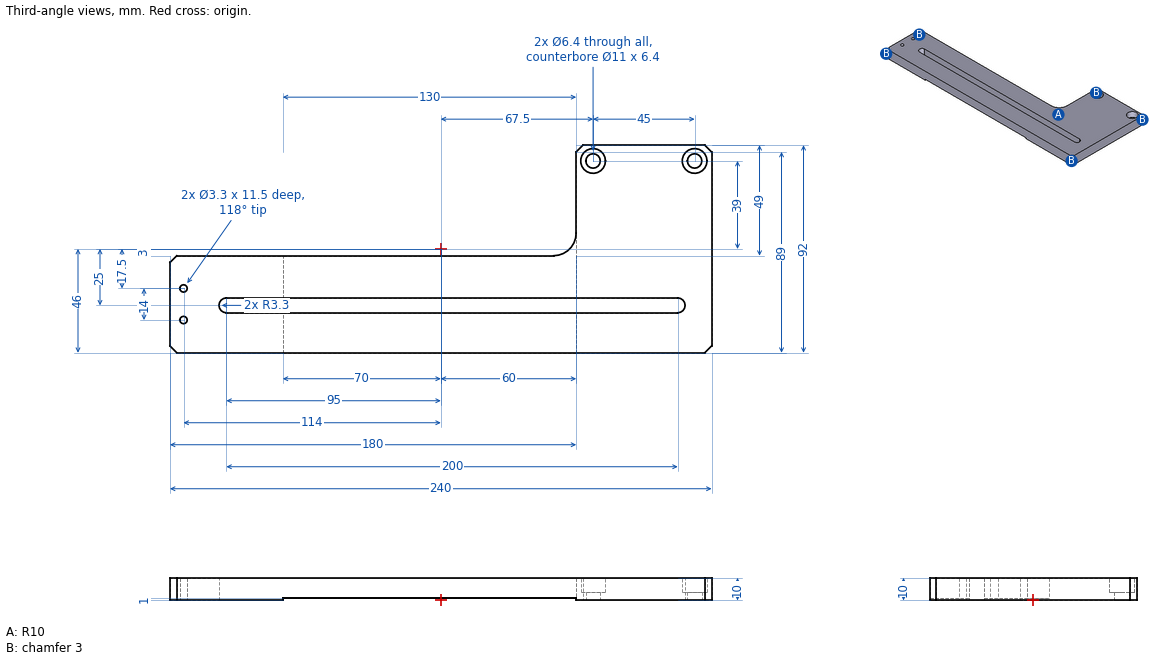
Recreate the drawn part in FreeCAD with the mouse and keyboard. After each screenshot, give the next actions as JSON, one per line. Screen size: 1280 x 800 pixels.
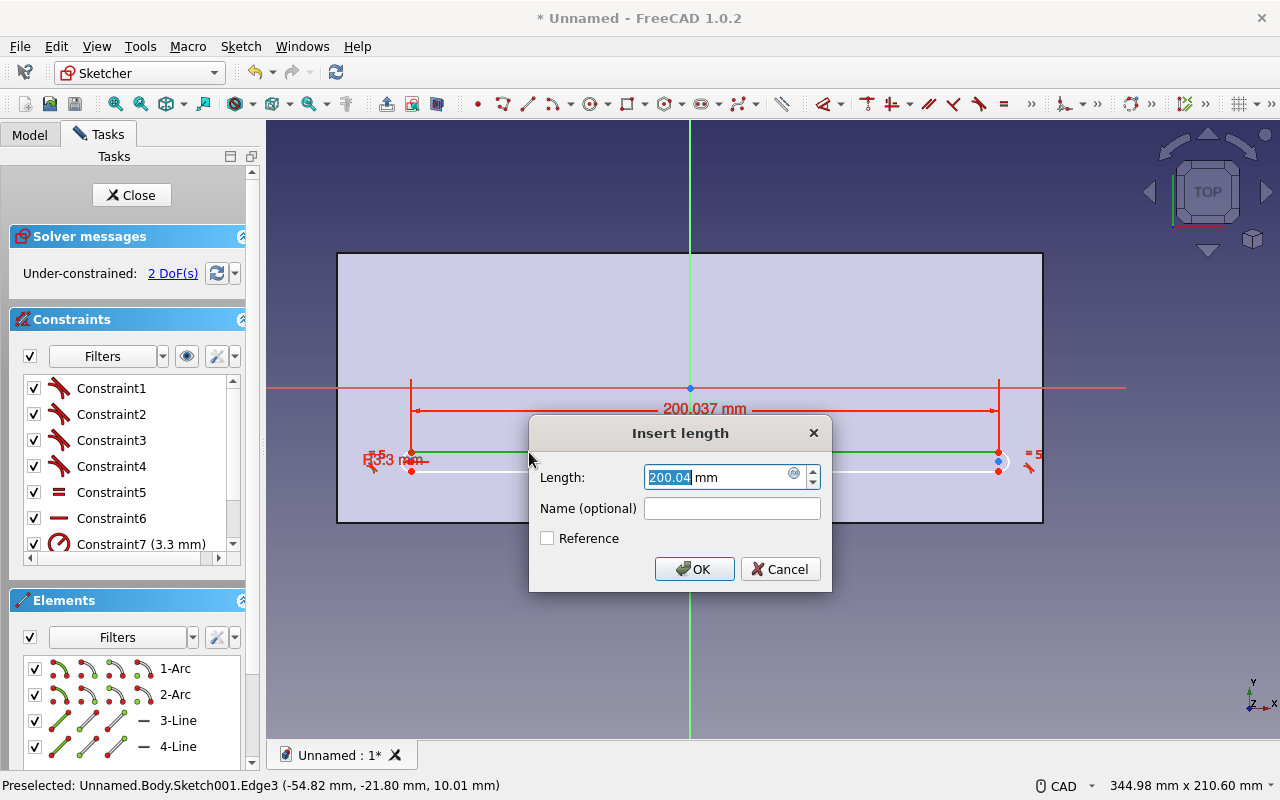
{"action": "type", "text": "200"}
{"action": "key", "text": "Return"}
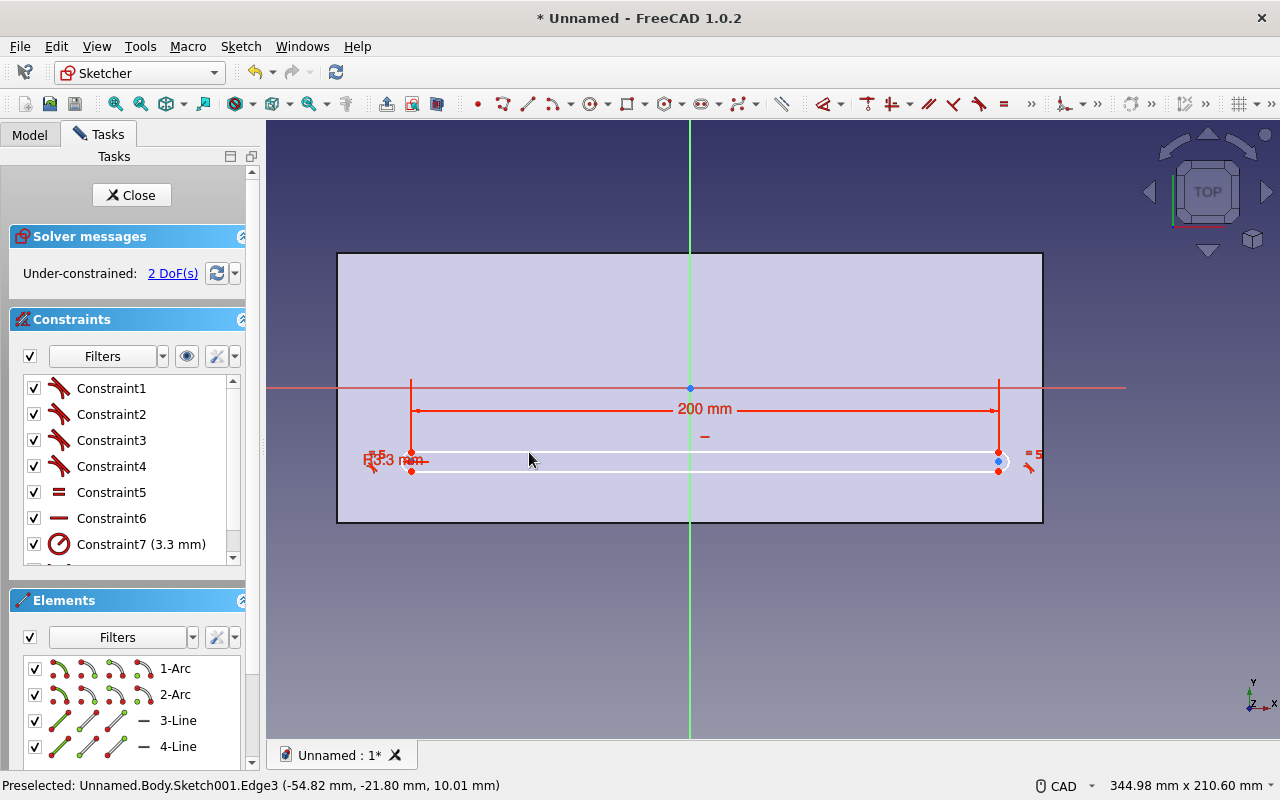
{"action": "scroll", "coordinate": [411, 452], "scroll_direction": "up", "scroll_amount": 2}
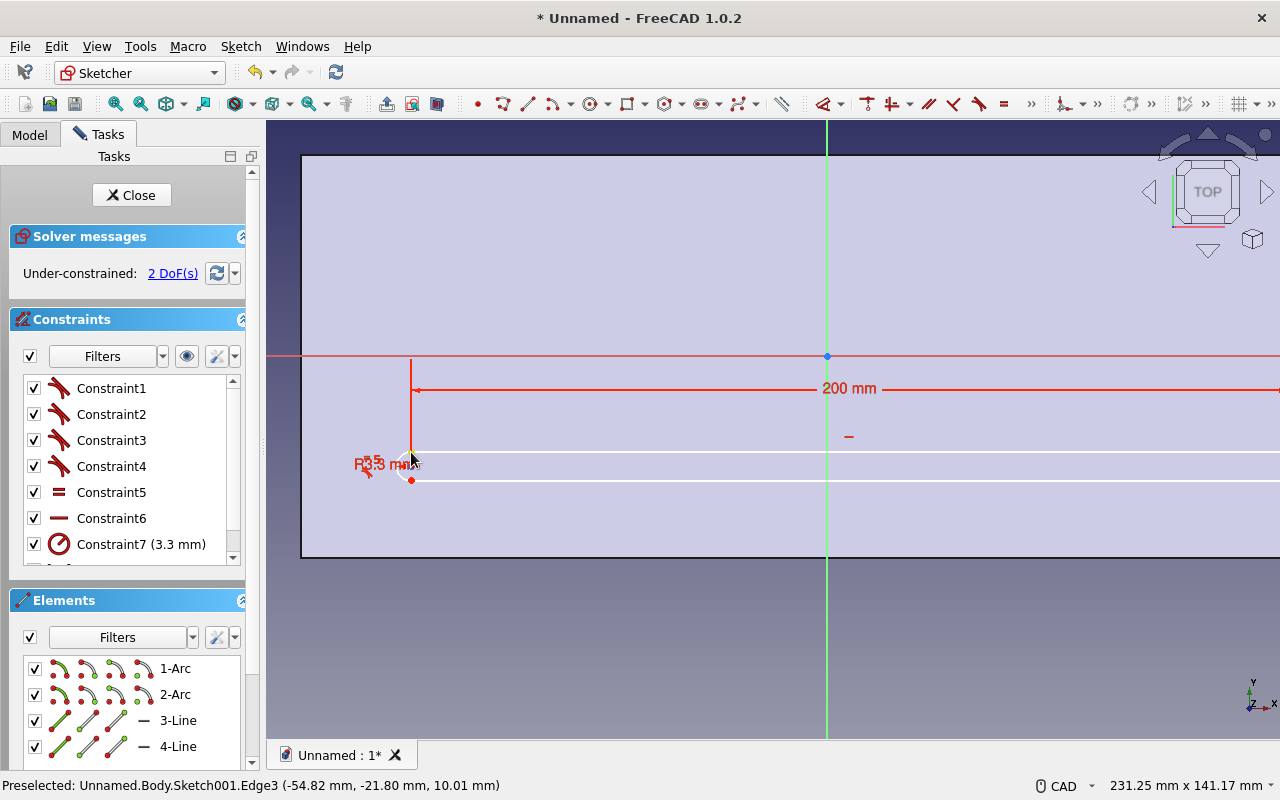
{"action": "left_click", "coordinate": [411, 452]}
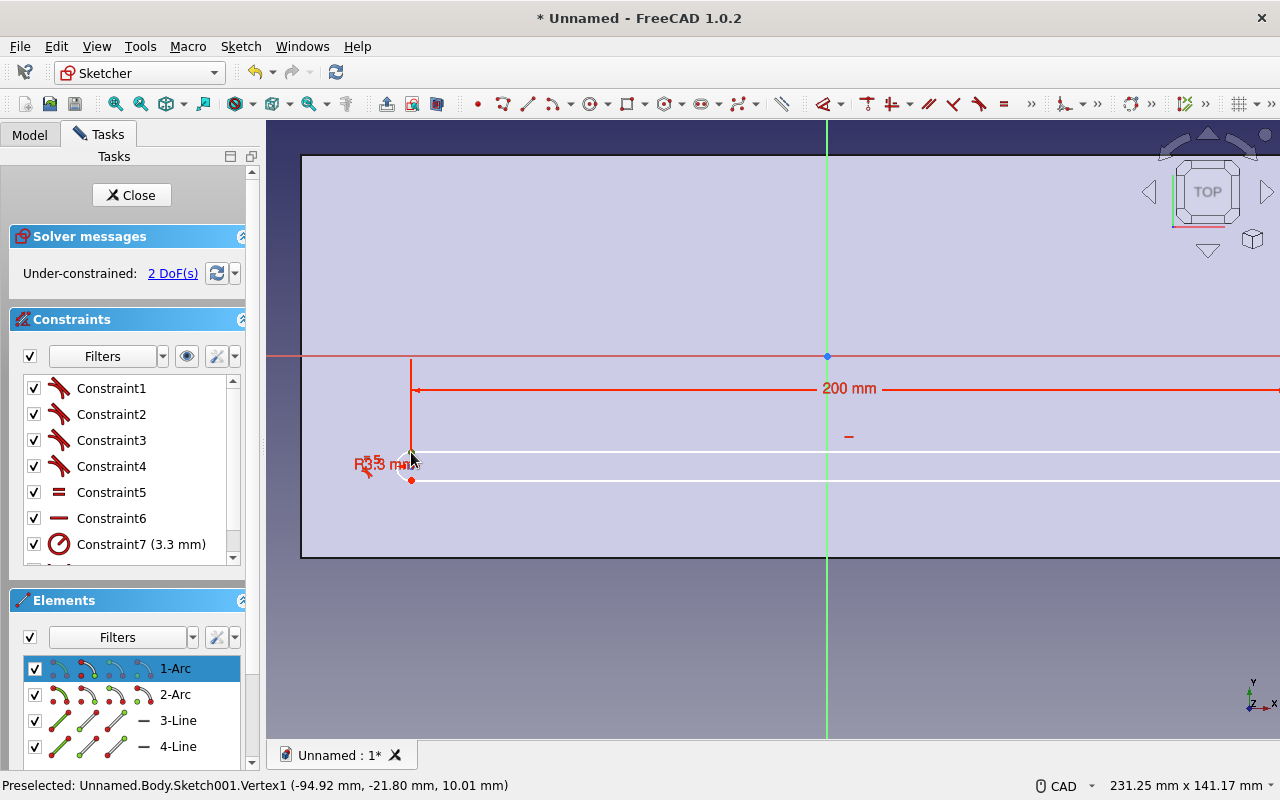
{"action": "key", "text": "l"}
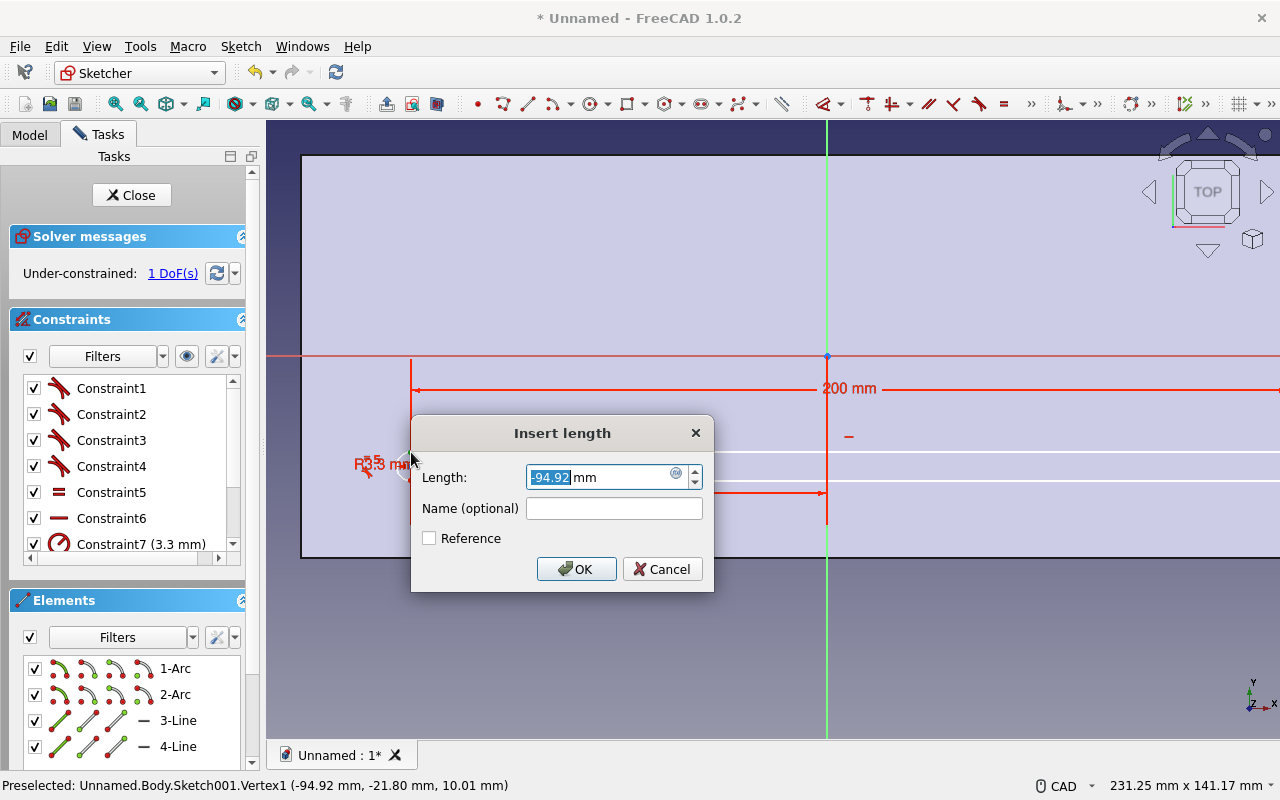
{"action": "type", "text": "-95"}
{"action": "key", "text": "Return"}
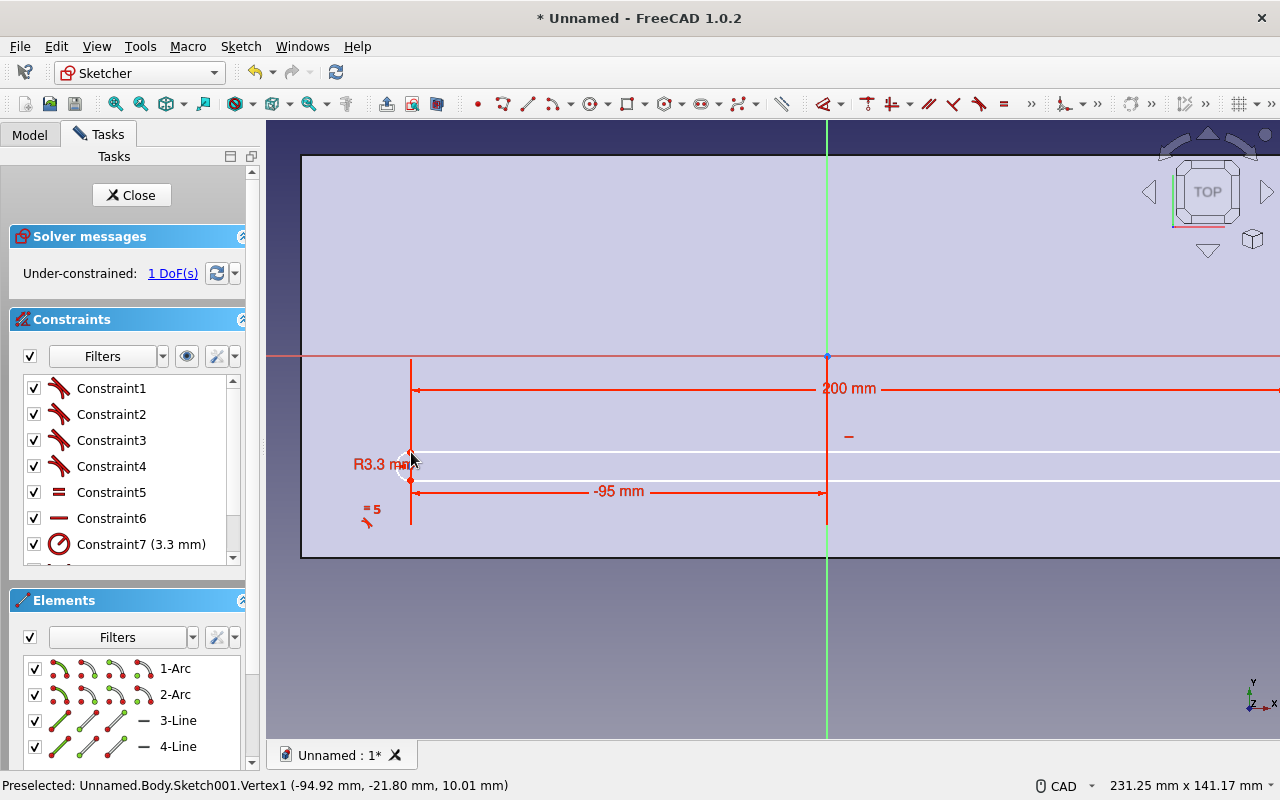
{"action": "left_click", "coordinate": [411, 466]}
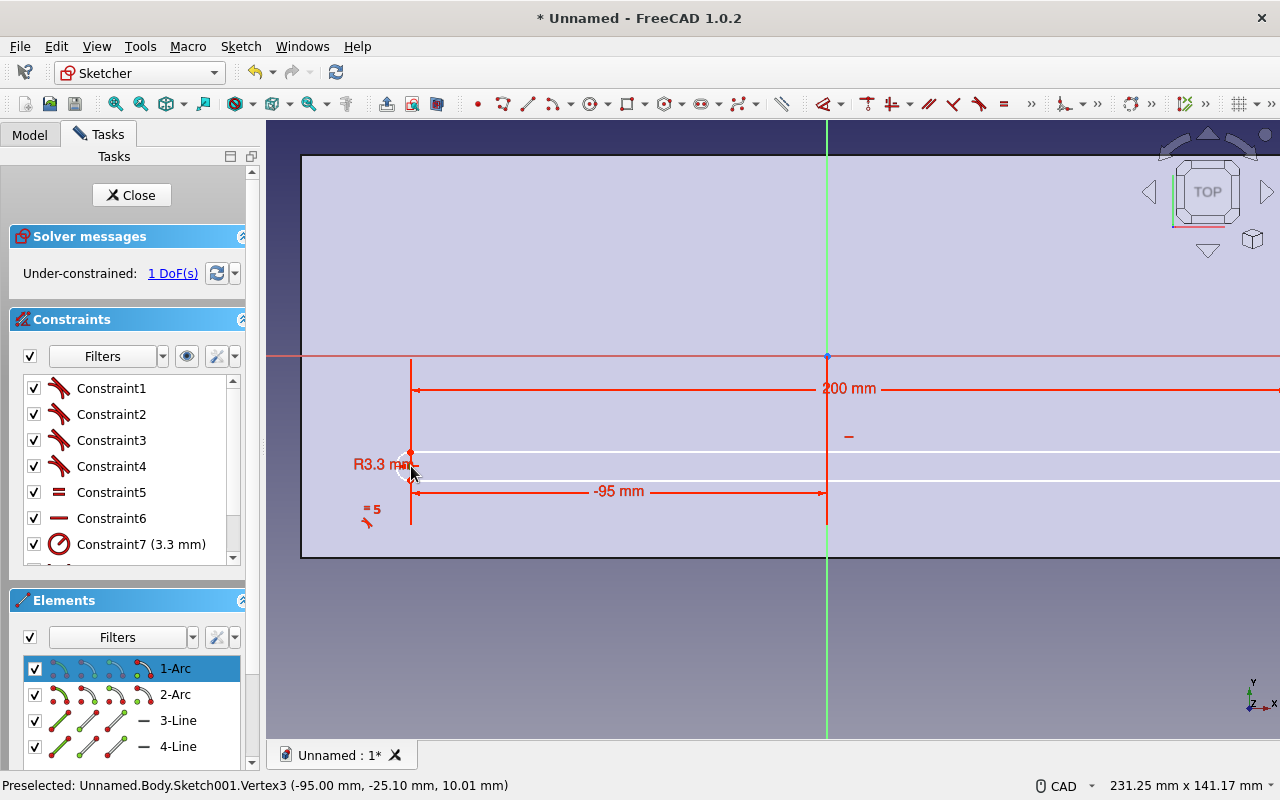
{"action": "key", "text": "i"}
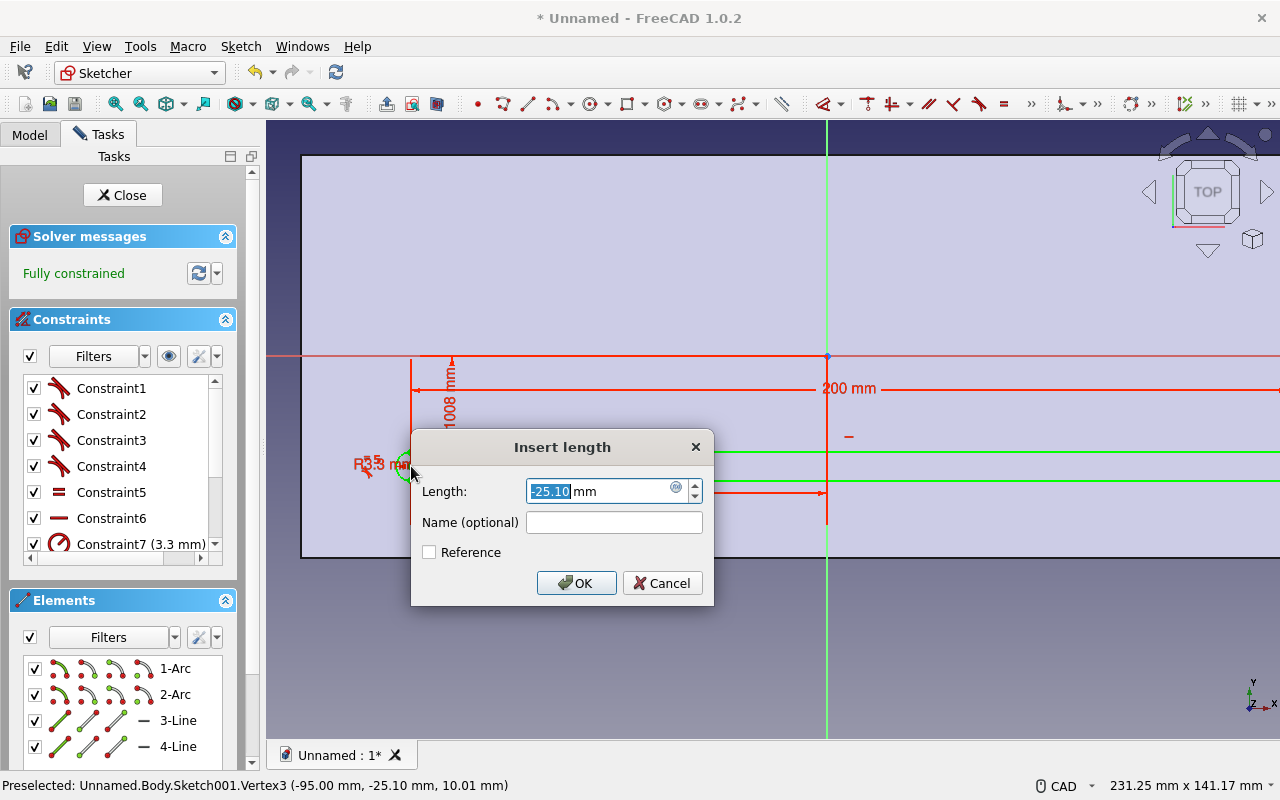
{"action": "type", "text": "-25"}
{"action": "key", "text": "Return"}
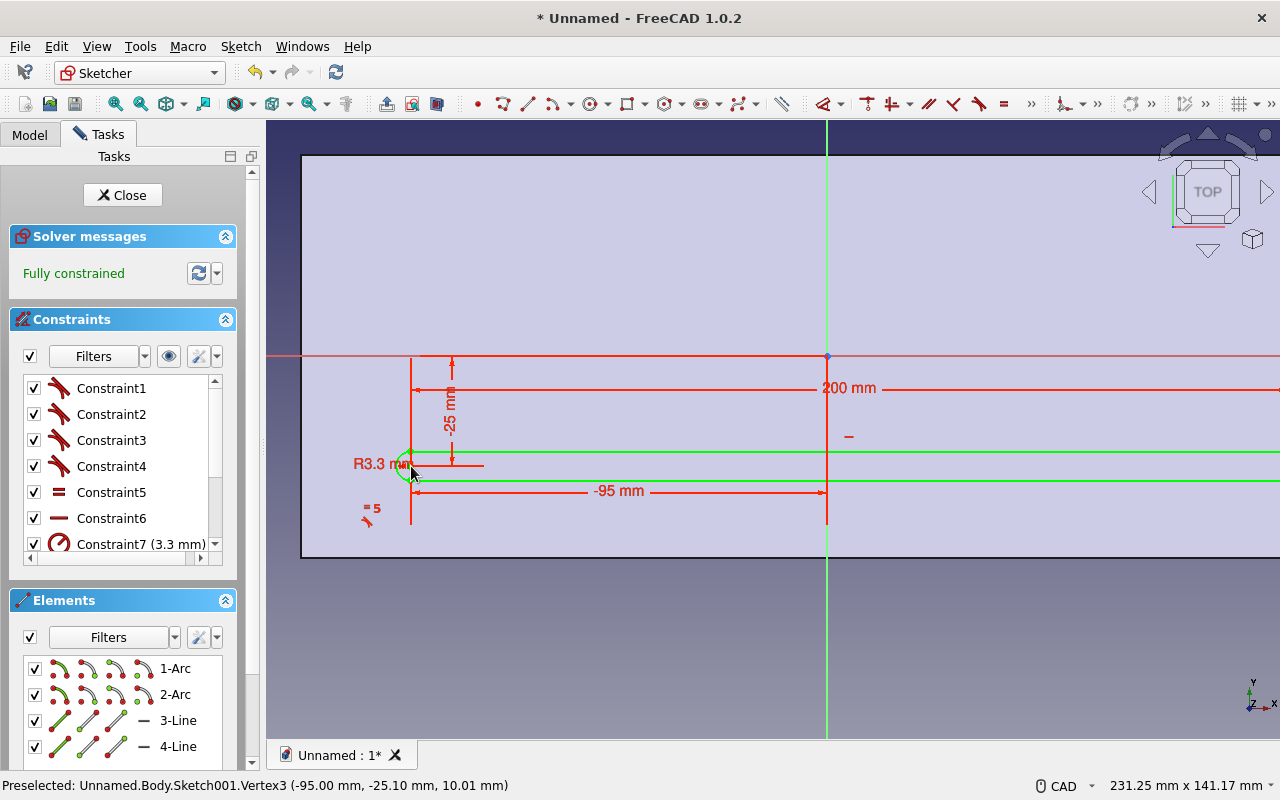
{"action": "left_click", "coordinate": [123, 195]}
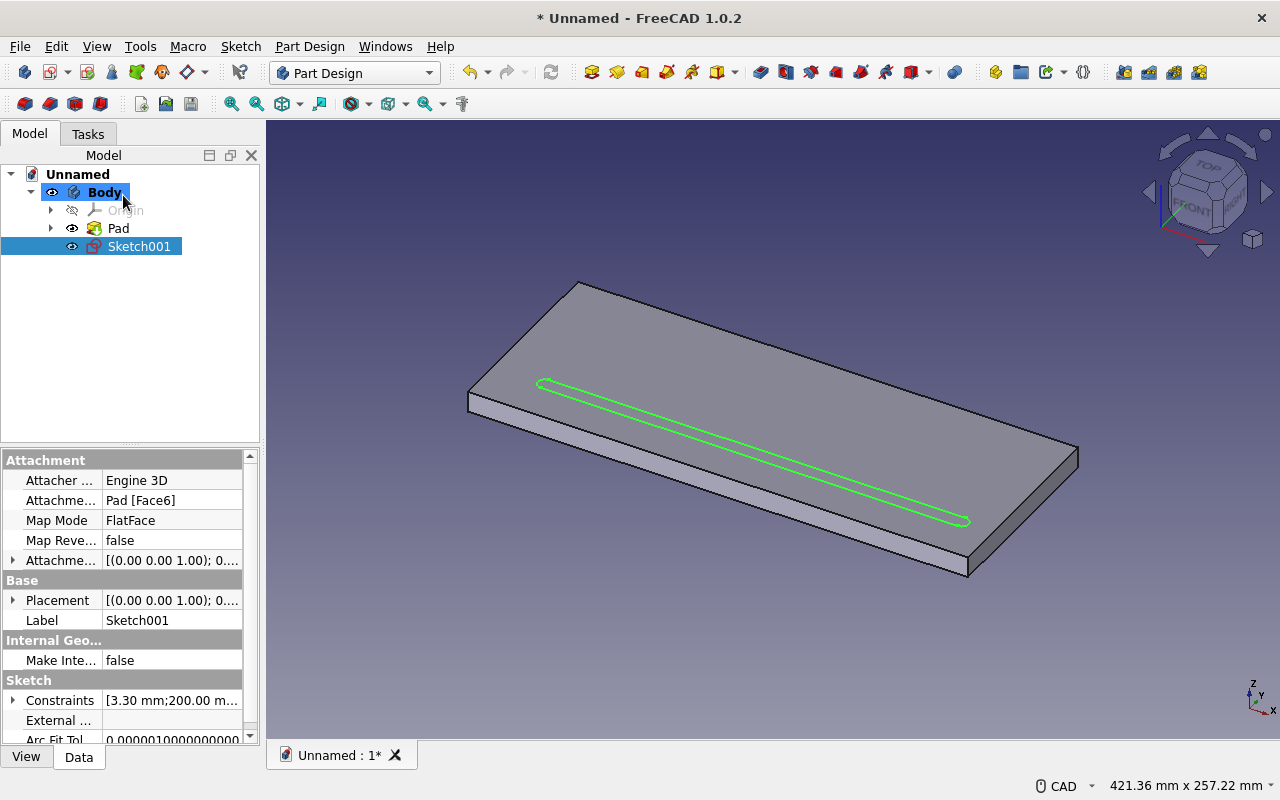
{"action": "left_click", "coordinate": [761, 72]}